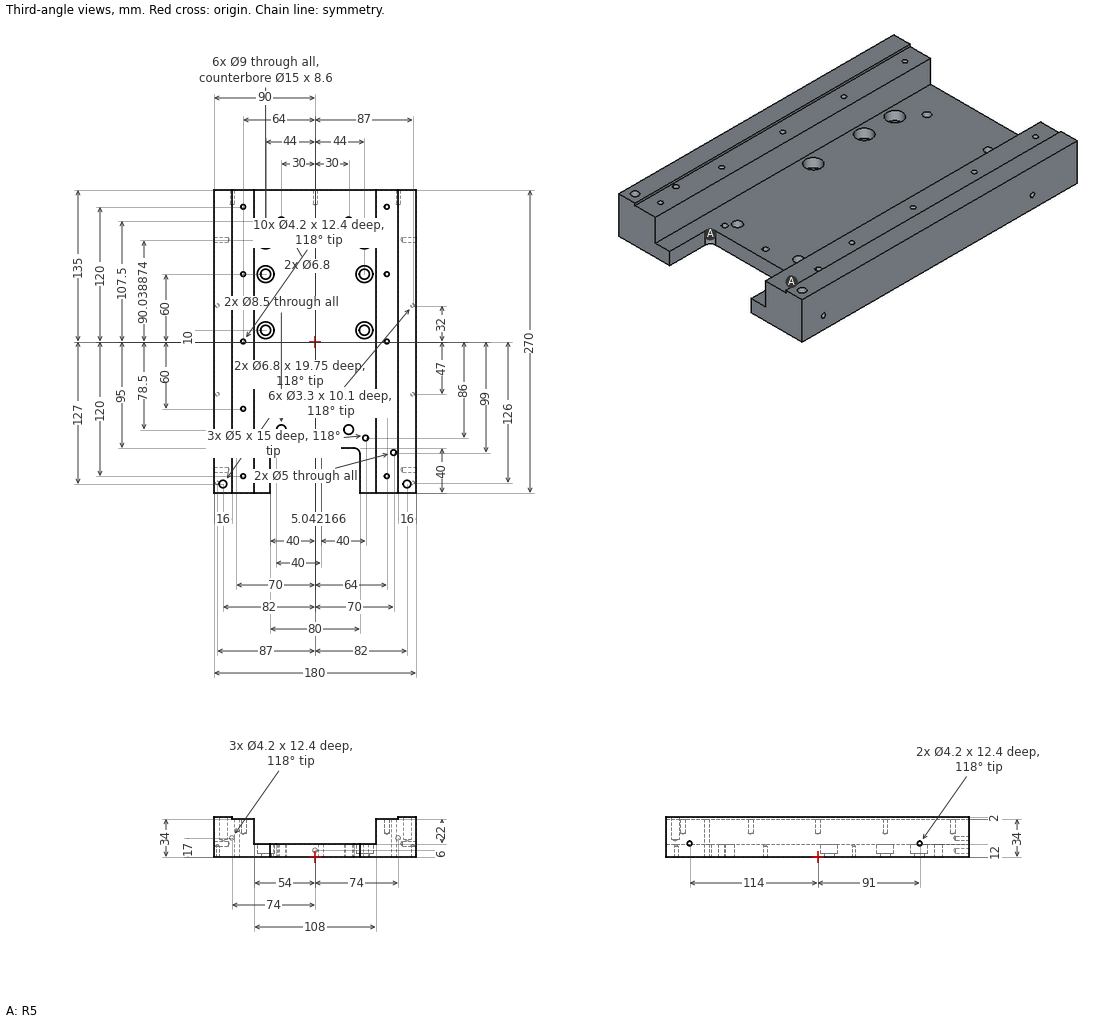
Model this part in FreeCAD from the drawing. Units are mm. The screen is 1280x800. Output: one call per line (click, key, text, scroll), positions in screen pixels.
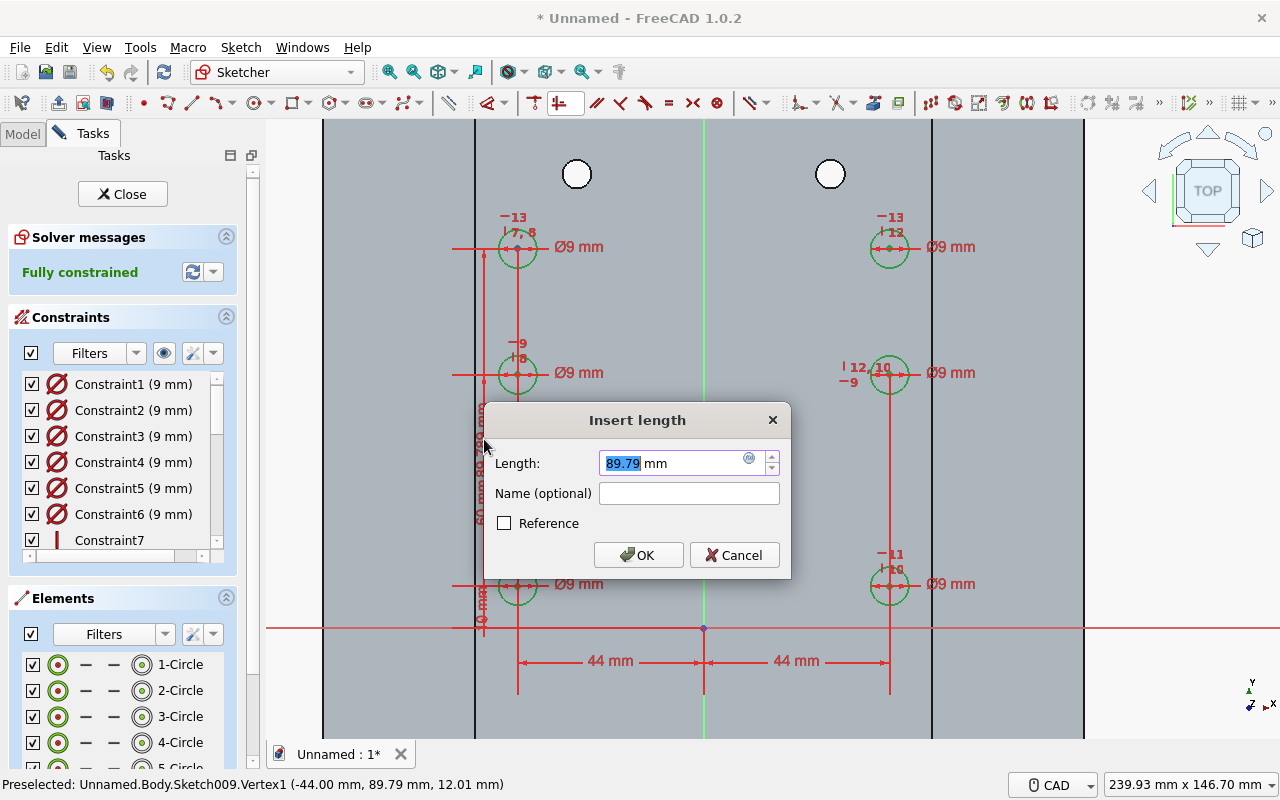
text(90.038874)
key(Return)
key(Escape)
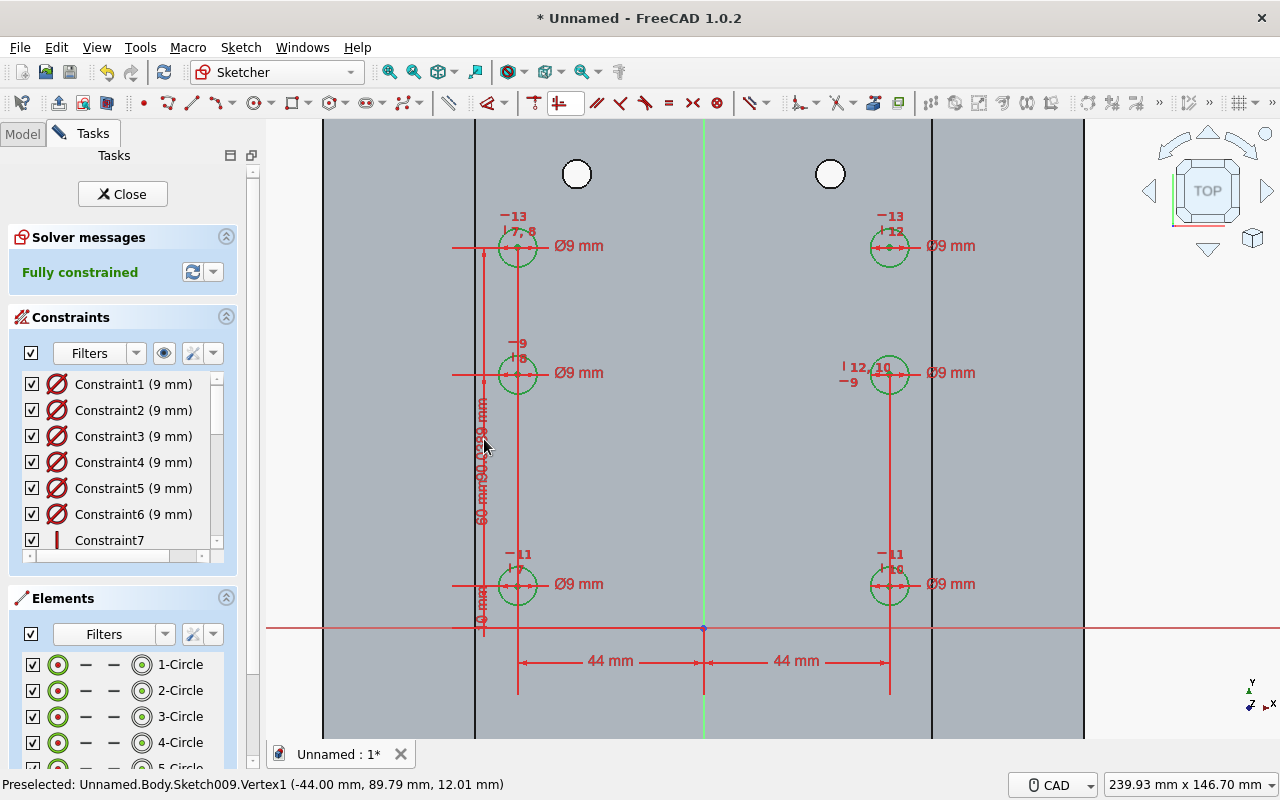
click(123, 194)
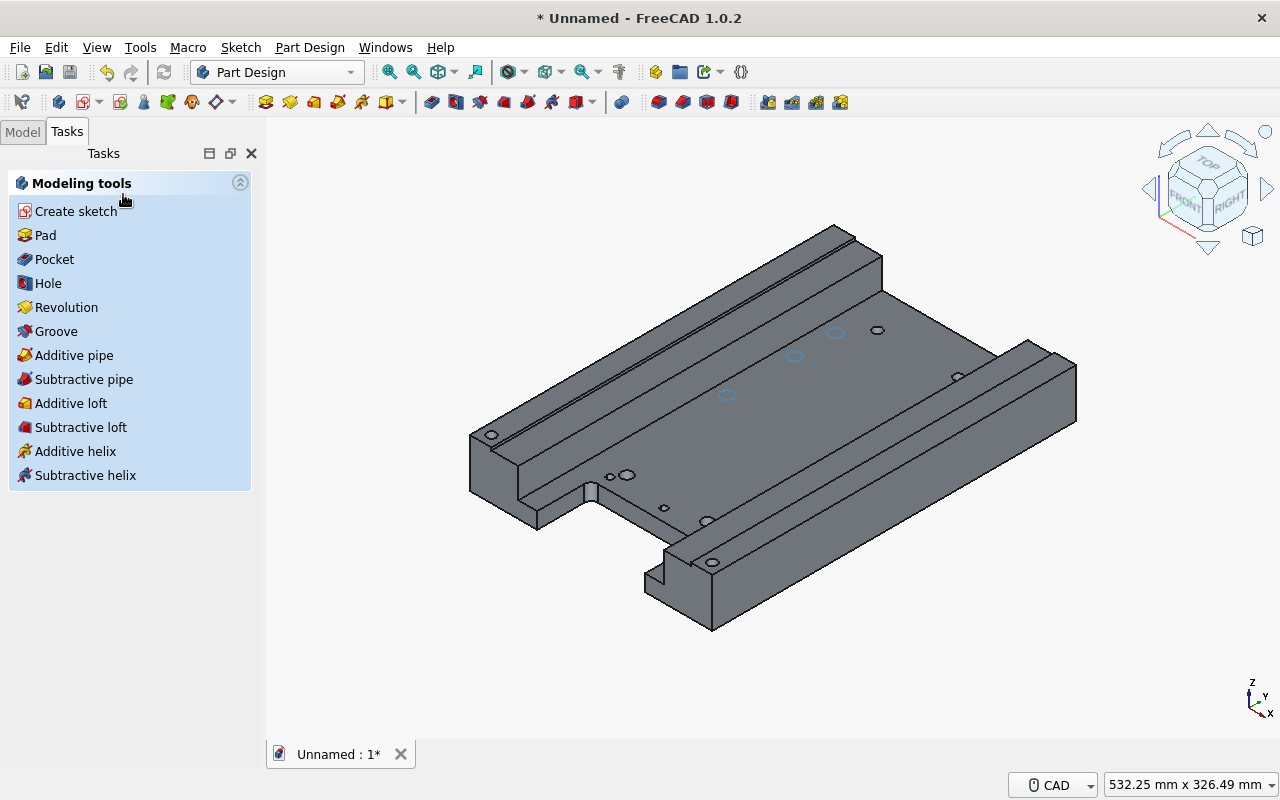
click(456, 102)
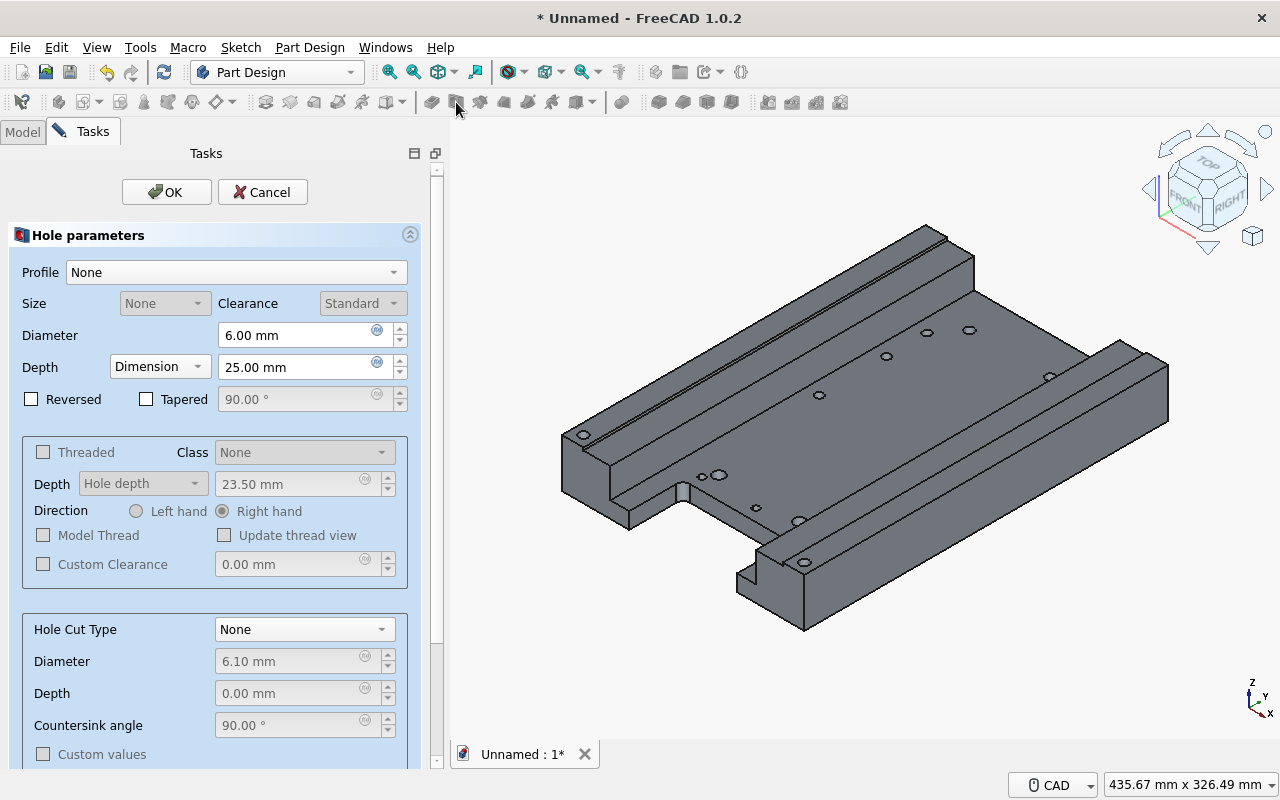
triple_click(305, 335)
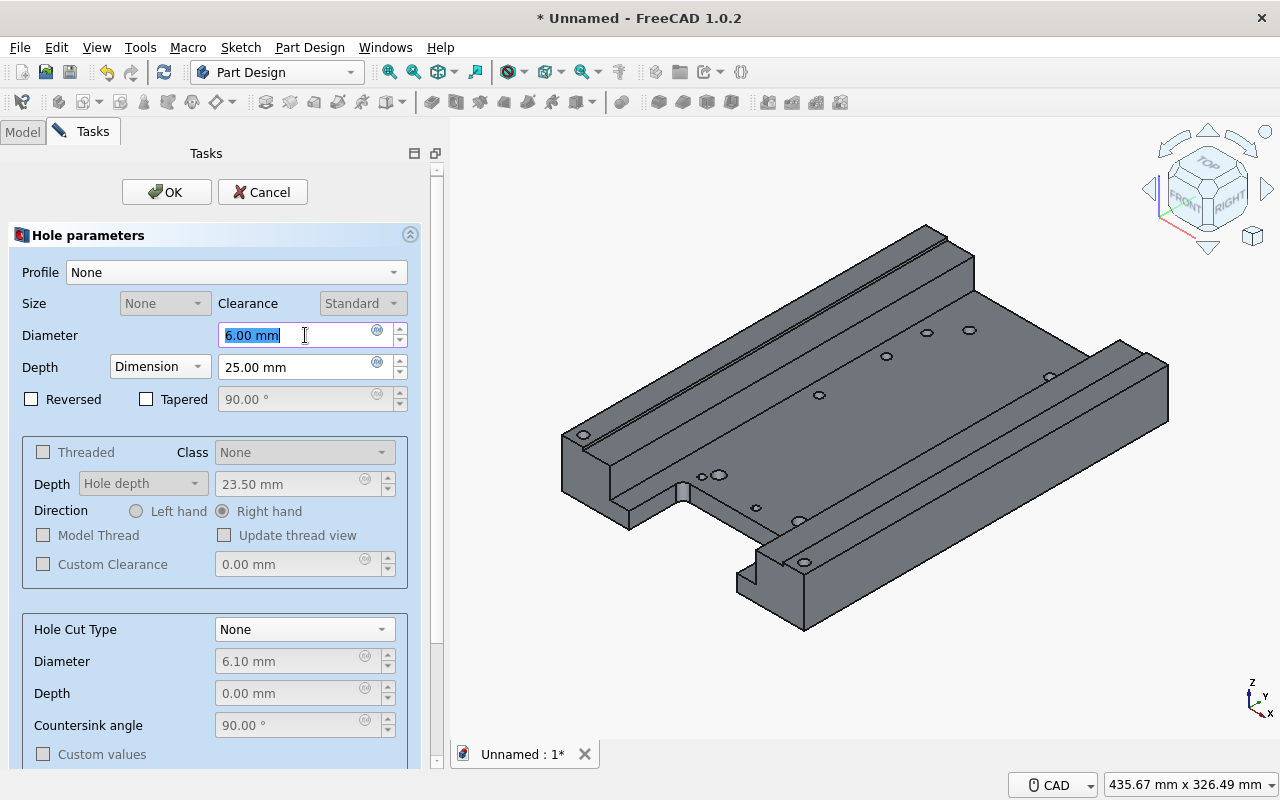
text(9)
key(Tab)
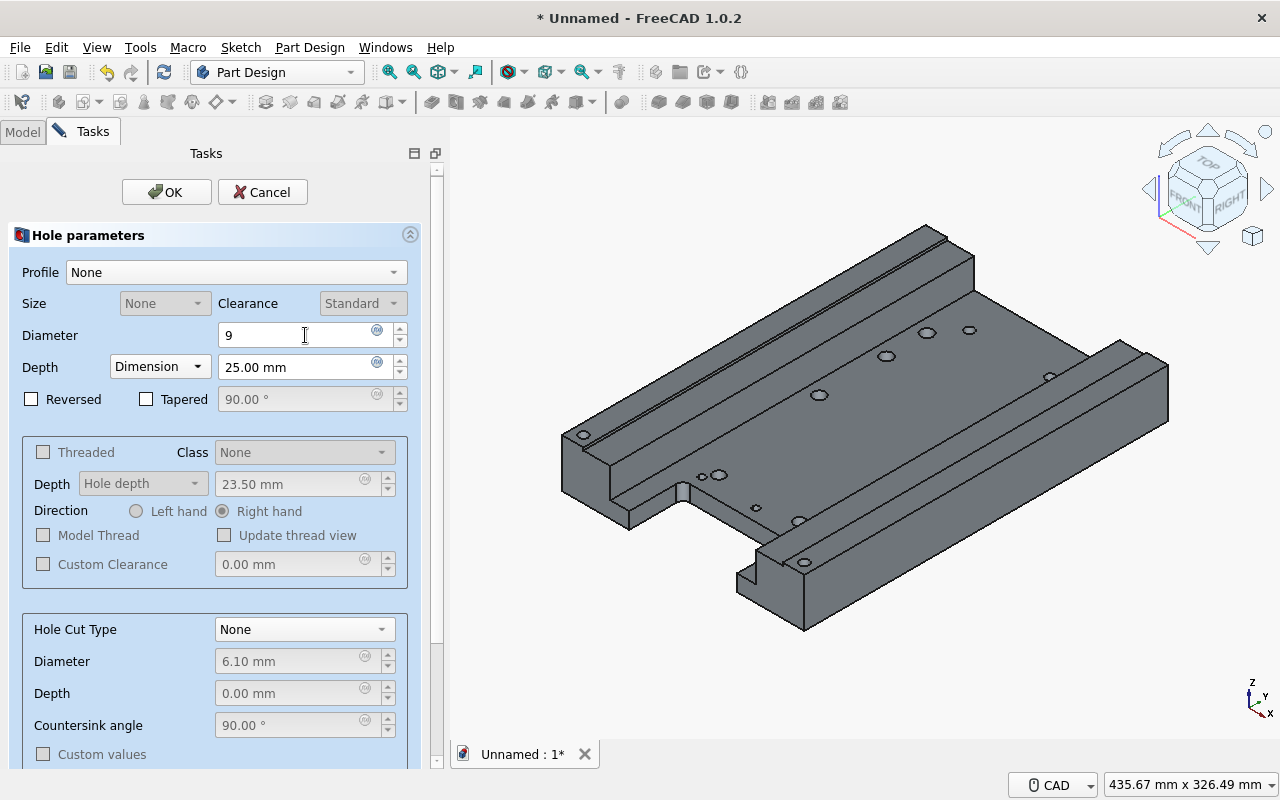
click(161, 366)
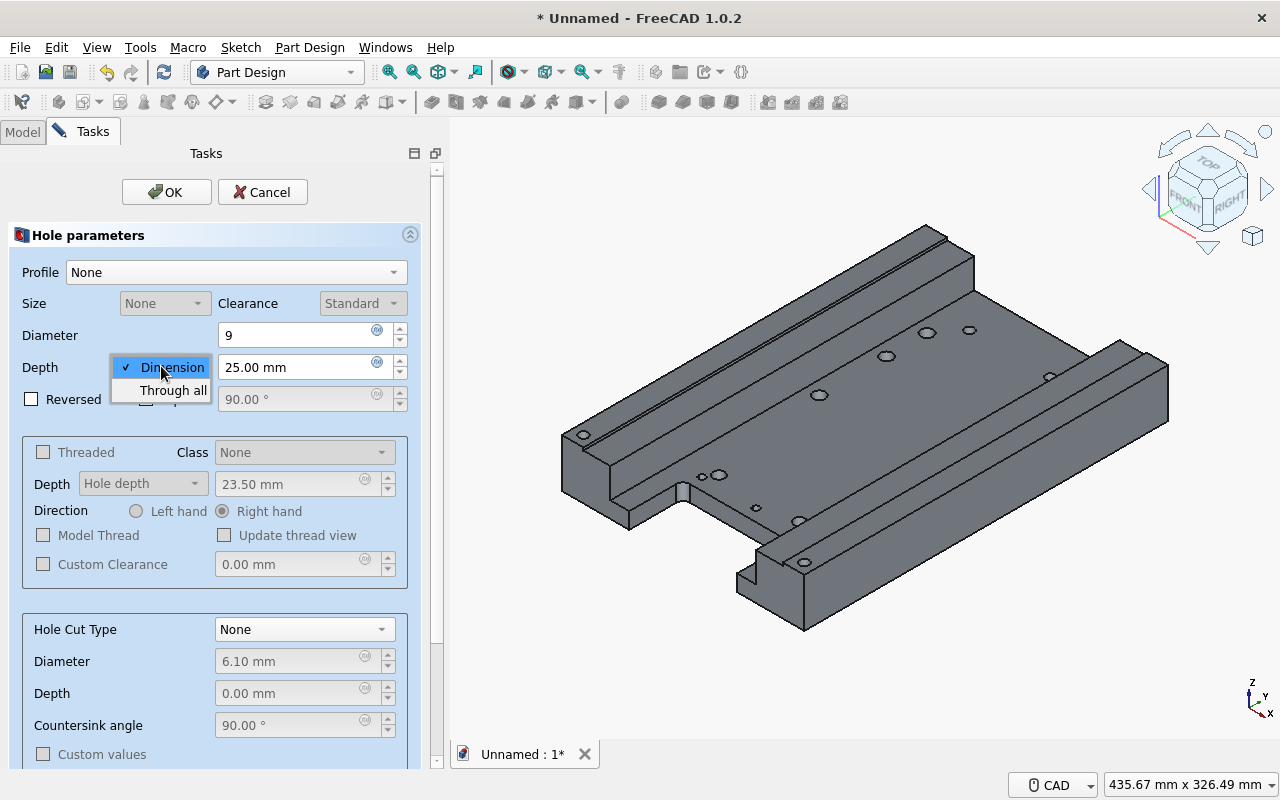
click(160, 390)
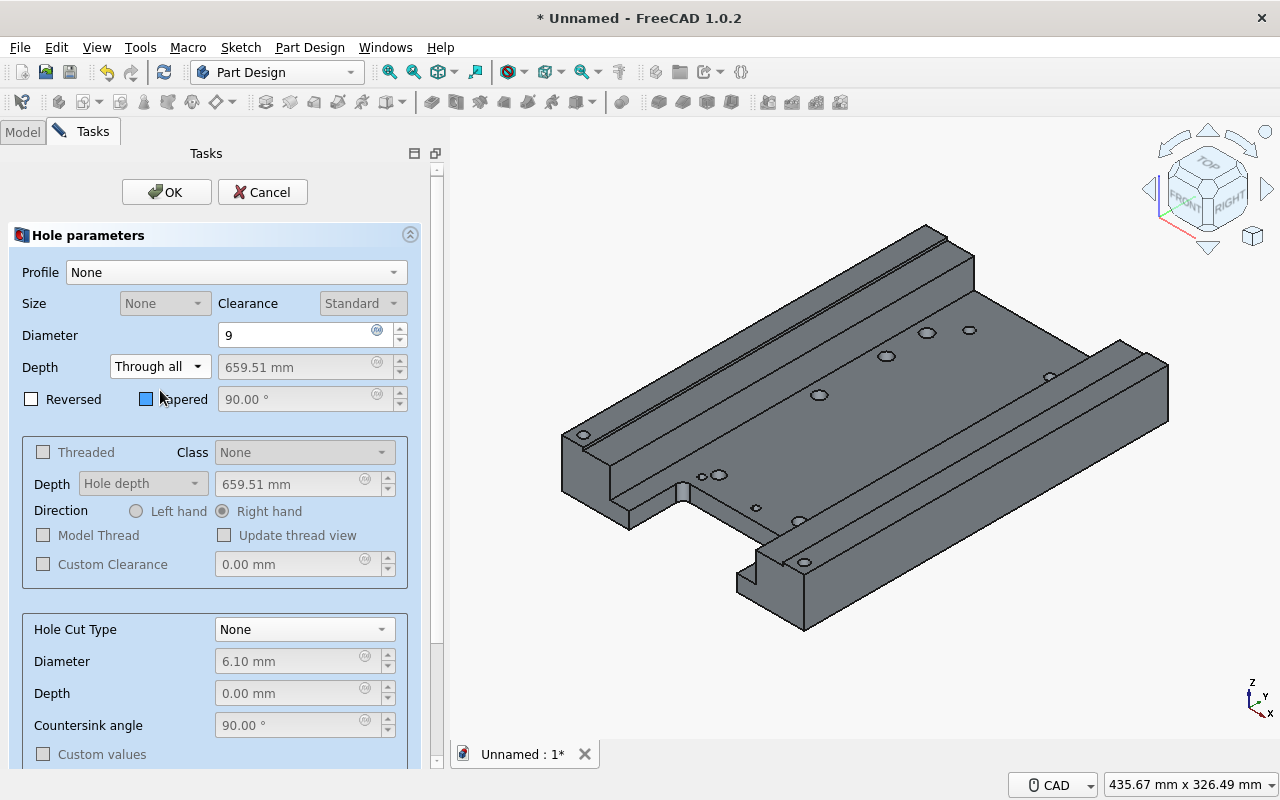
click(306, 630)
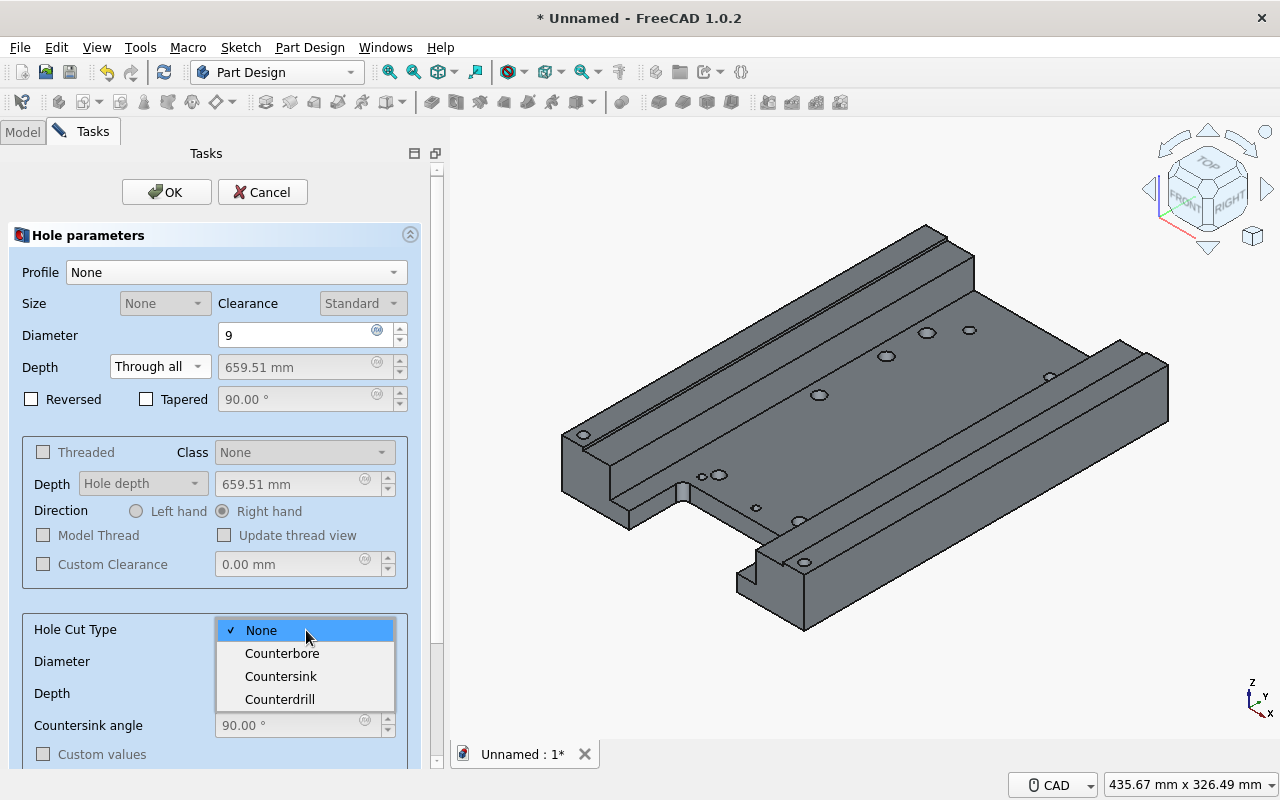
click(304, 654)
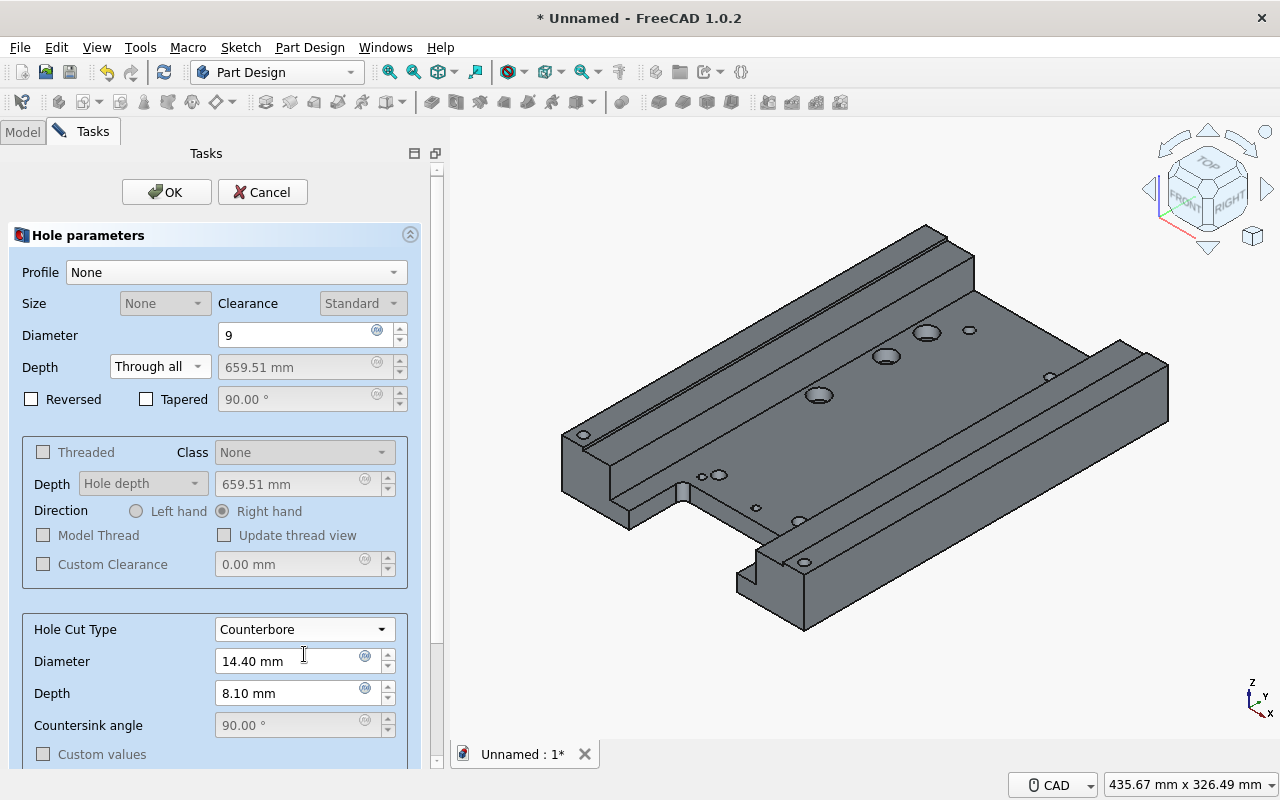
triple_click(298, 661)